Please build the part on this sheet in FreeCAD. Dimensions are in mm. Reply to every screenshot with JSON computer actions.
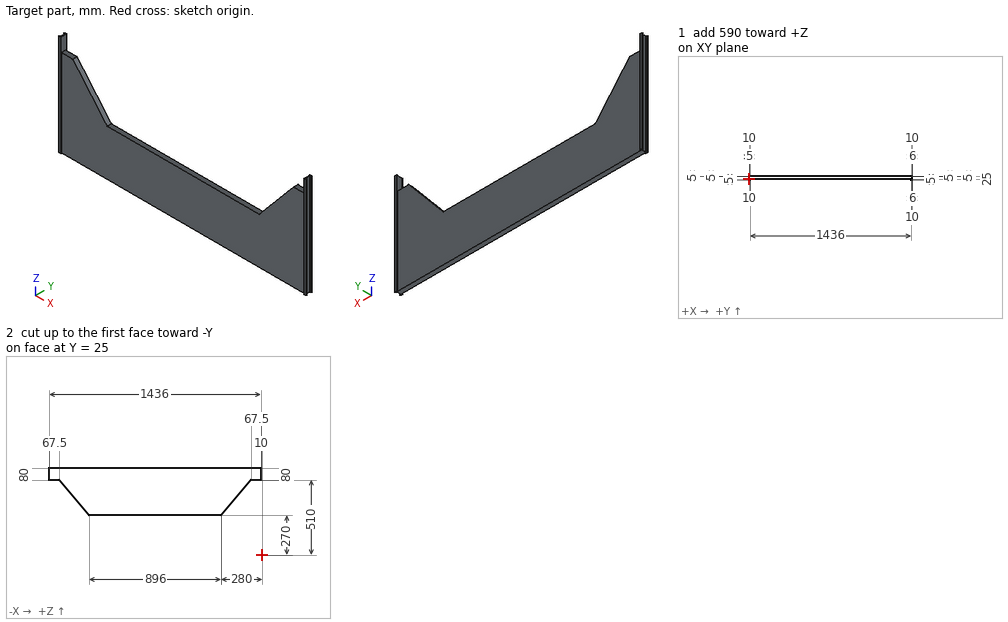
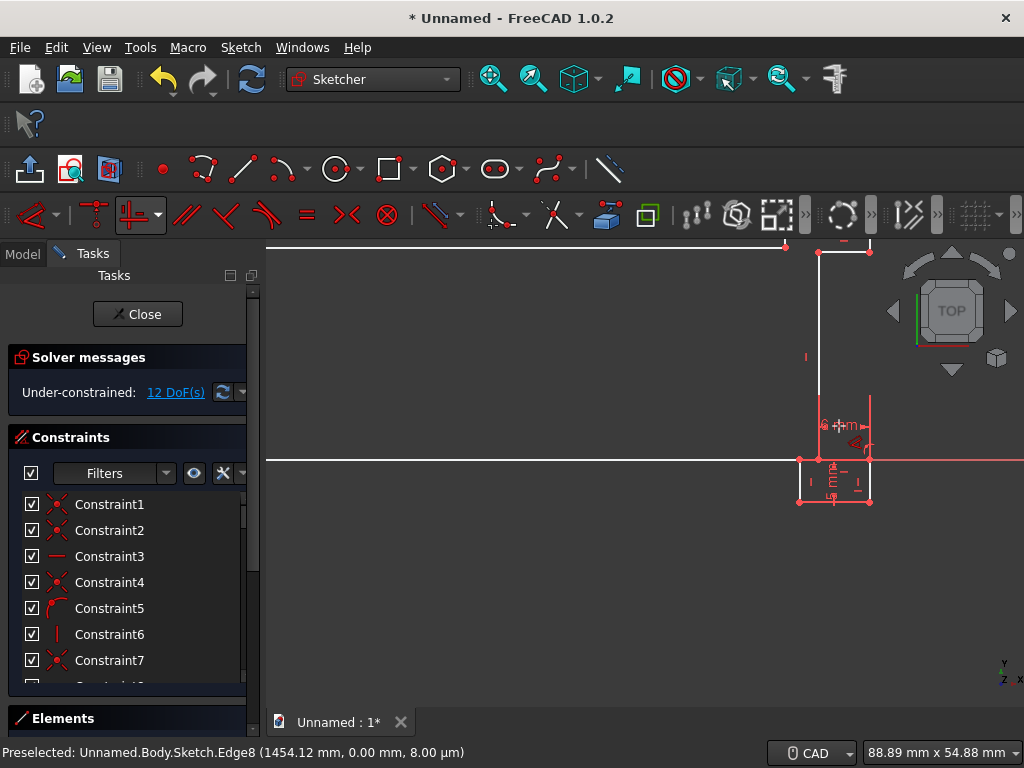
{"action": "scroll", "coordinate": [828, 478], "scroll_direction": "down", "scroll_amount": 16}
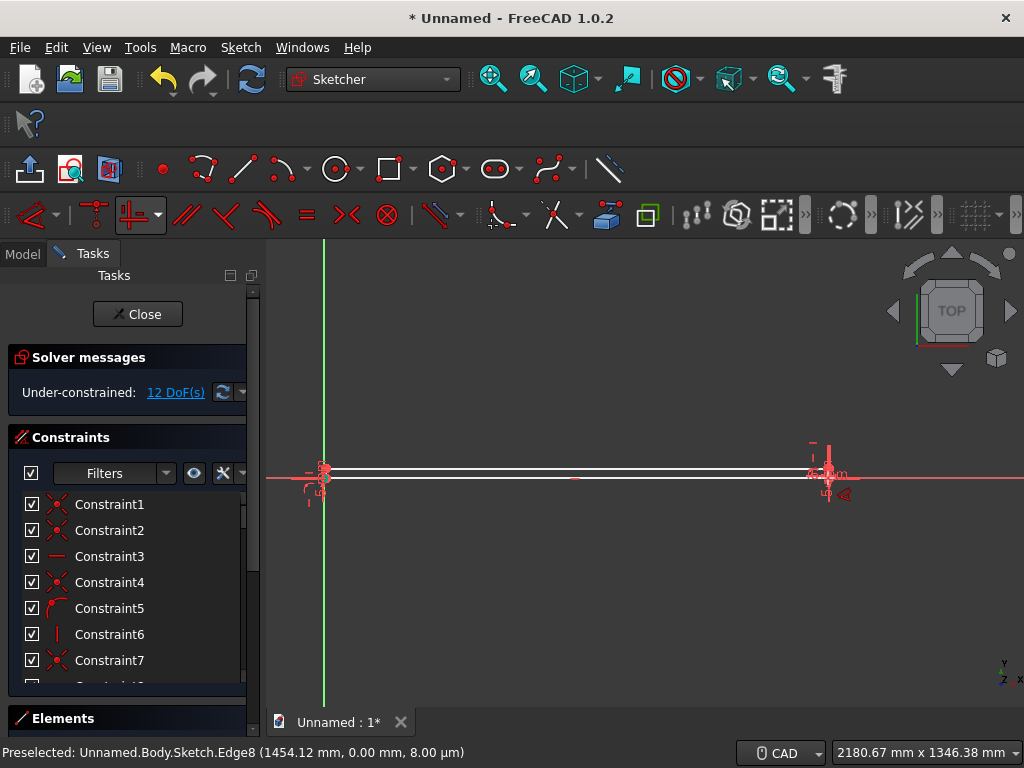
{"action": "scroll", "coordinate": [829, 469], "scroll_direction": "up", "scroll_amount": 15}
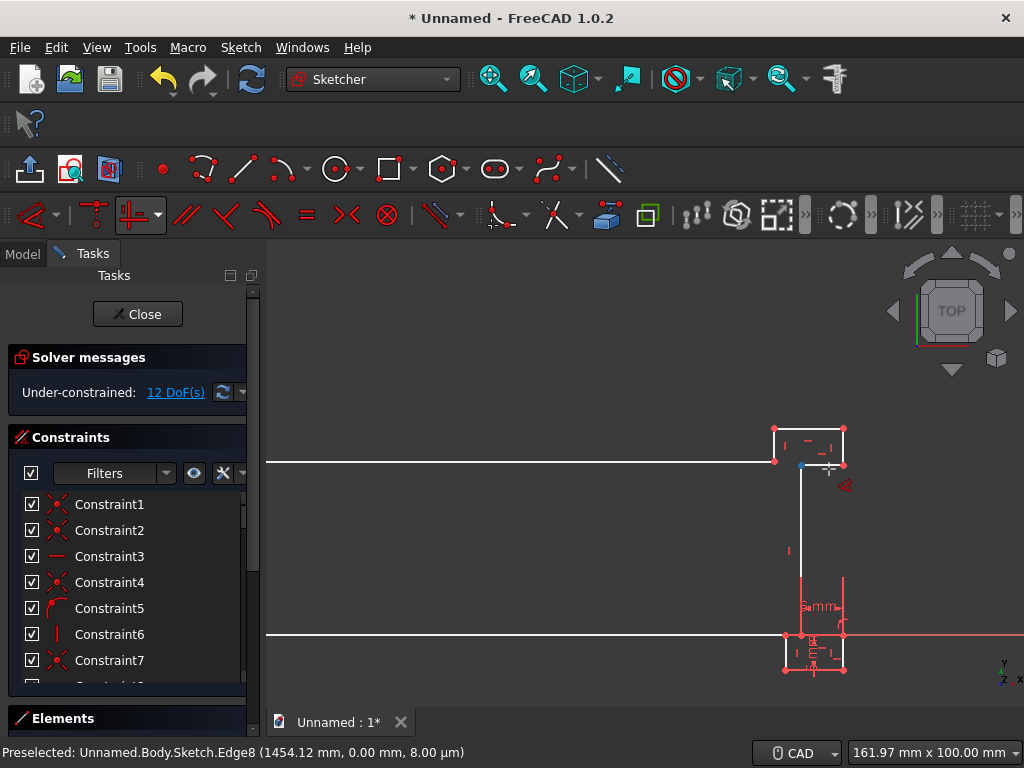
{"action": "left_click", "coordinate": [814, 465]}
{"action": "left_click", "coordinate": [822, 499]}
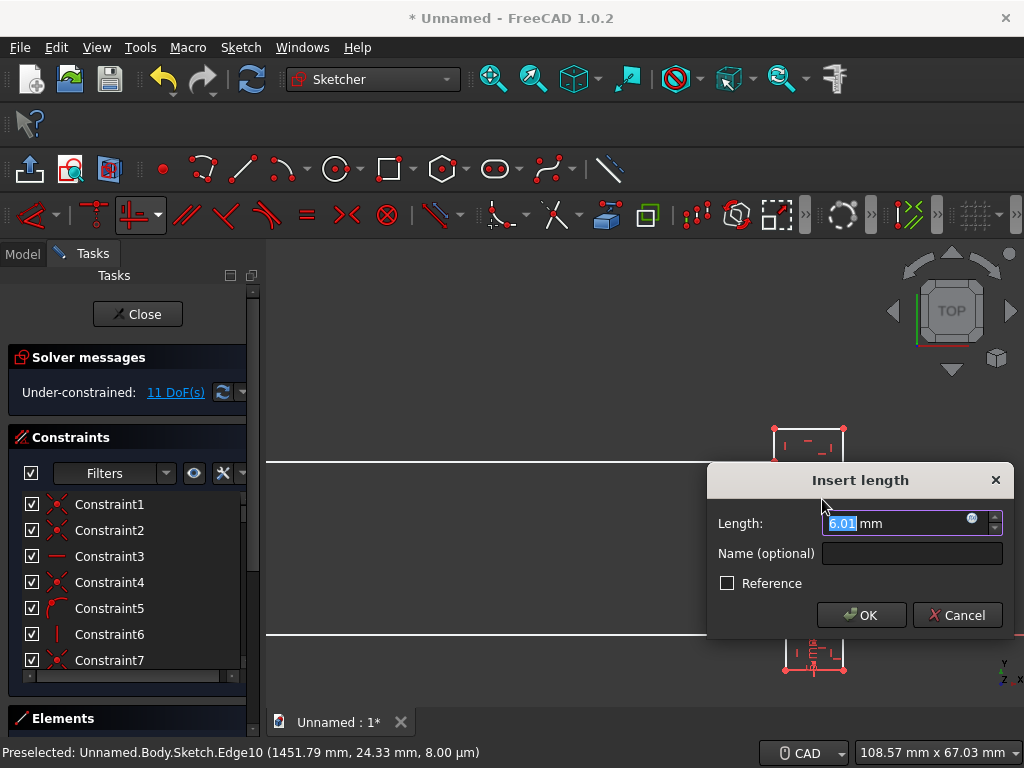
{"action": "type", "text": "6"}
{"action": "key", "text": "Return"}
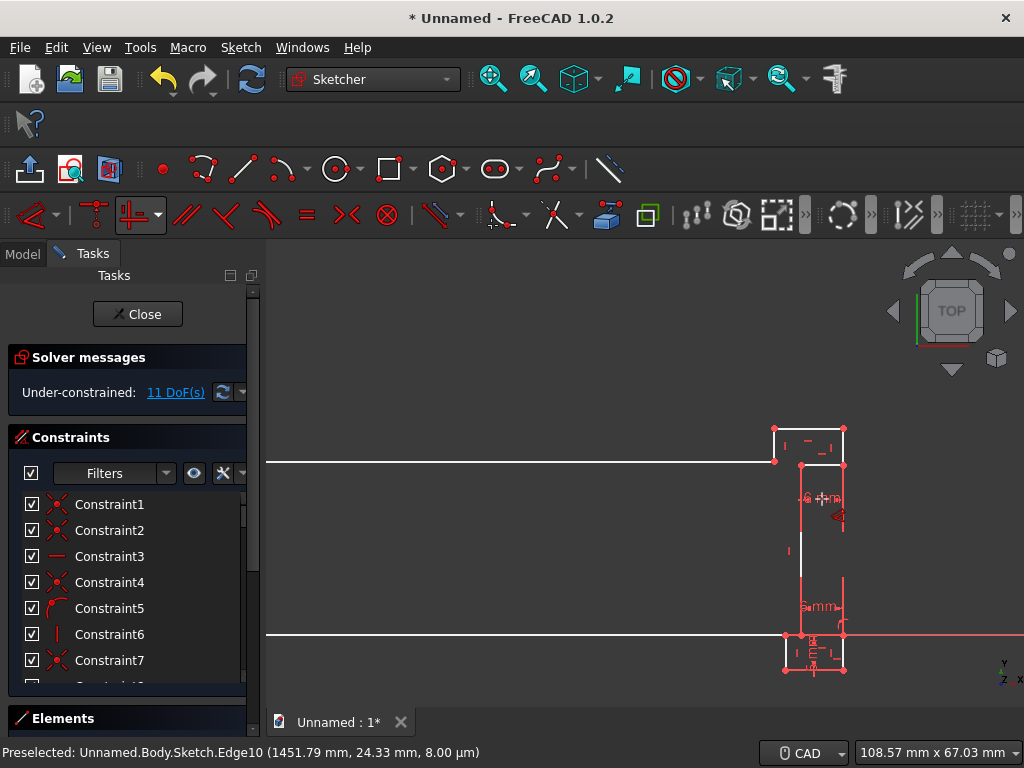
{"action": "left_click", "coordinate": [843, 454]}
{"action": "left_click", "coordinate": [809, 447]}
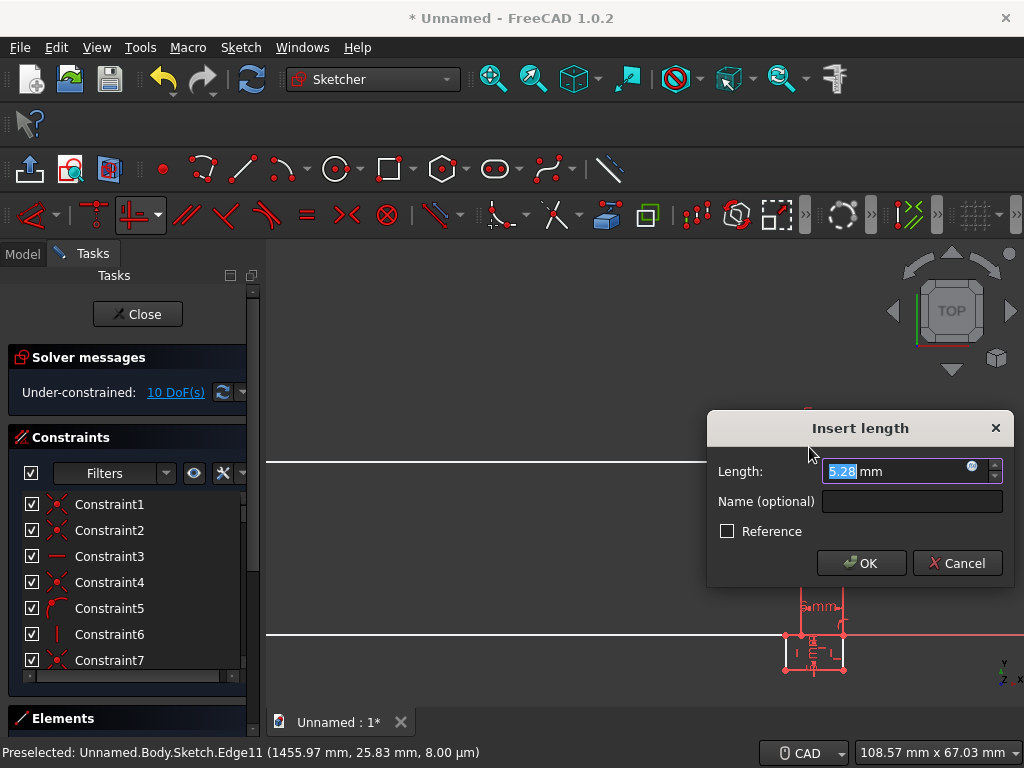
{"action": "type", "text": "5"}
{"action": "key", "text": "Return"}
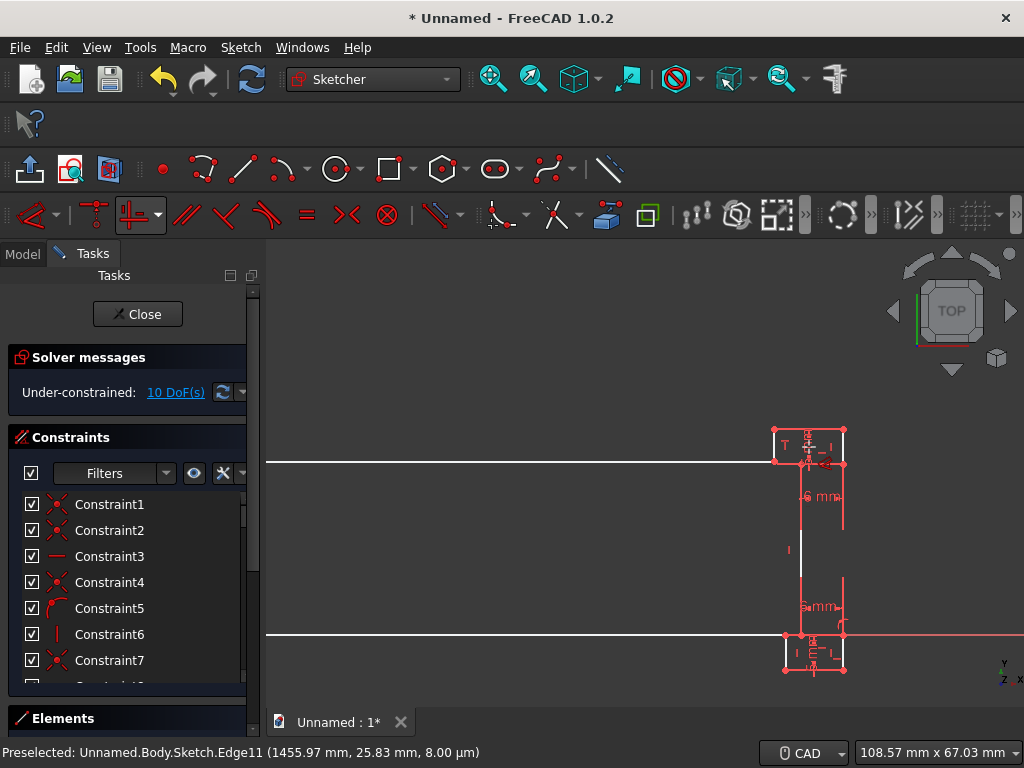
{"action": "left_click", "coordinate": [774, 439]}
{"action": "left_click", "coordinate": [716, 445]}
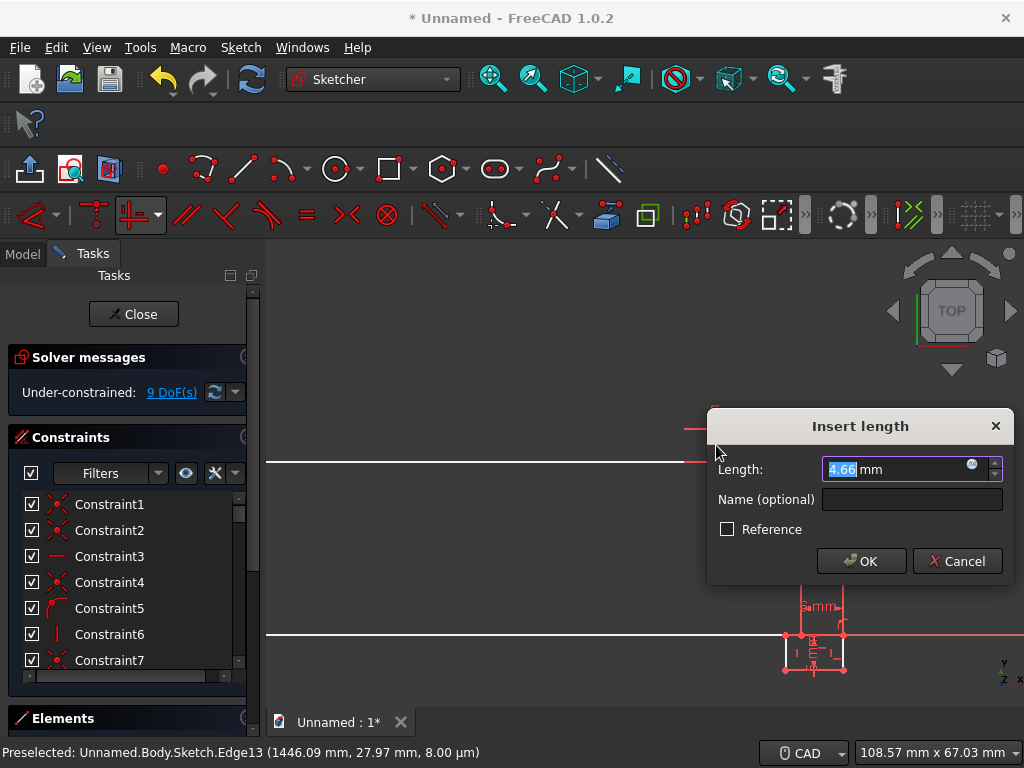
{"action": "type", "text": "5"}
{"action": "key", "text": "Return"}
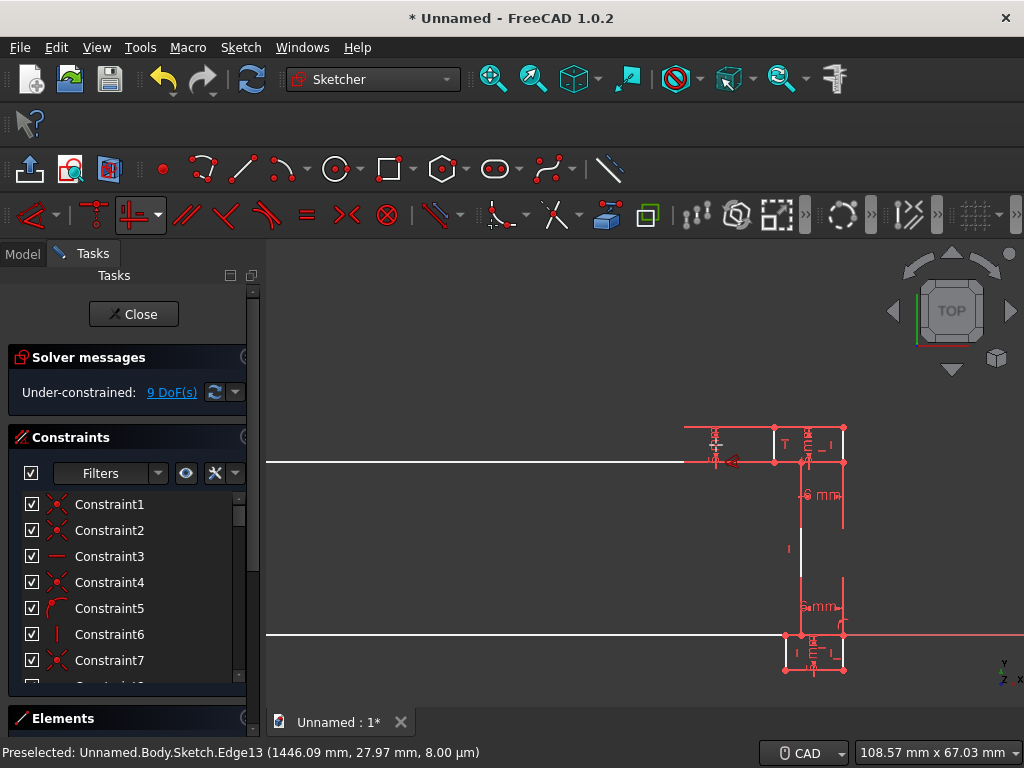
{"action": "scroll", "coordinate": [829, 469], "scroll_direction": "down", "scroll_amount": 15}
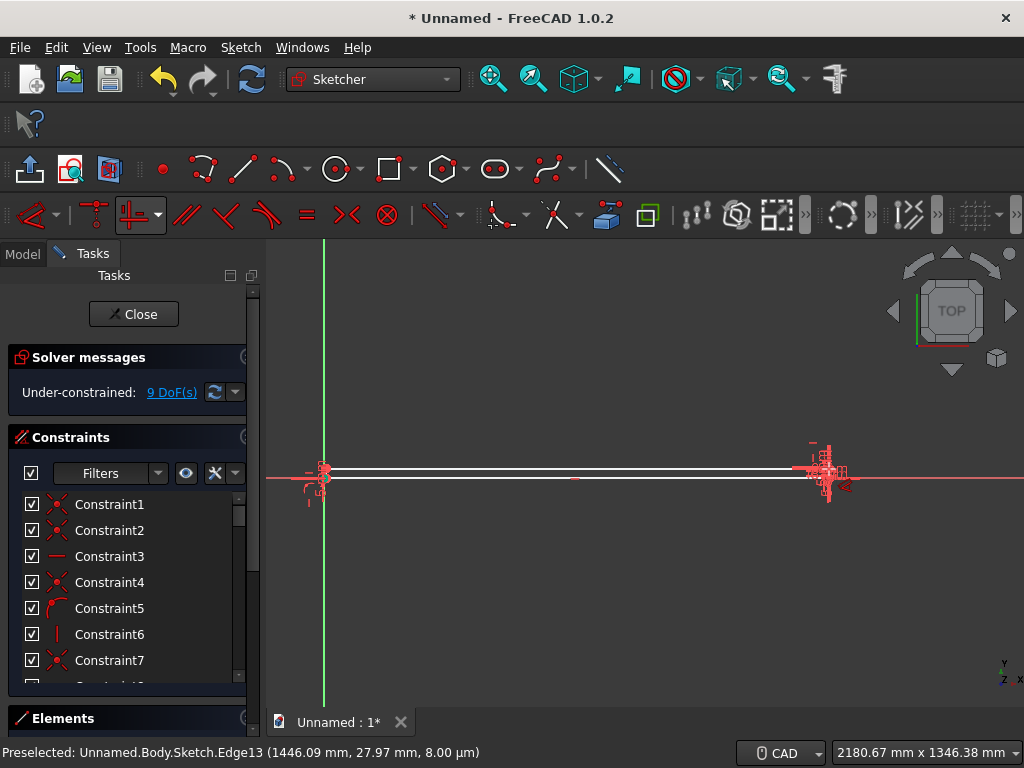
{"action": "scroll", "coordinate": [328, 469], "scroll_direction": "up", "scroll_amount": 16}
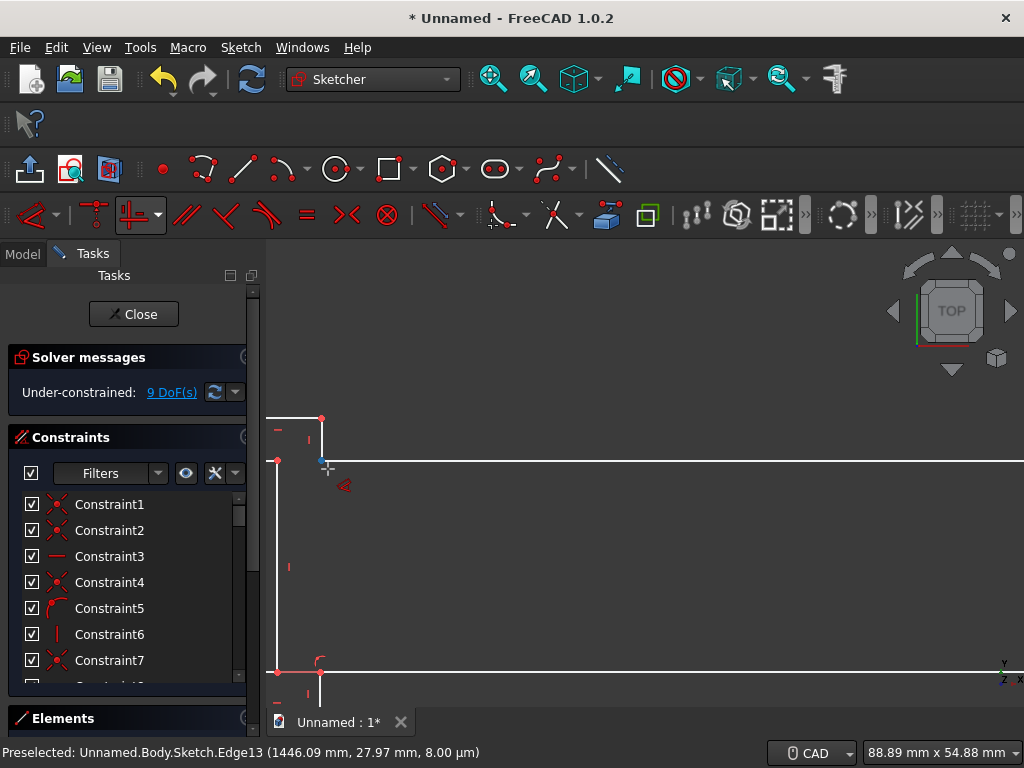
{"action": "left_click", "coordinate": [322, 448]}
{"action": "left_click", "coordinate": [356, 439]}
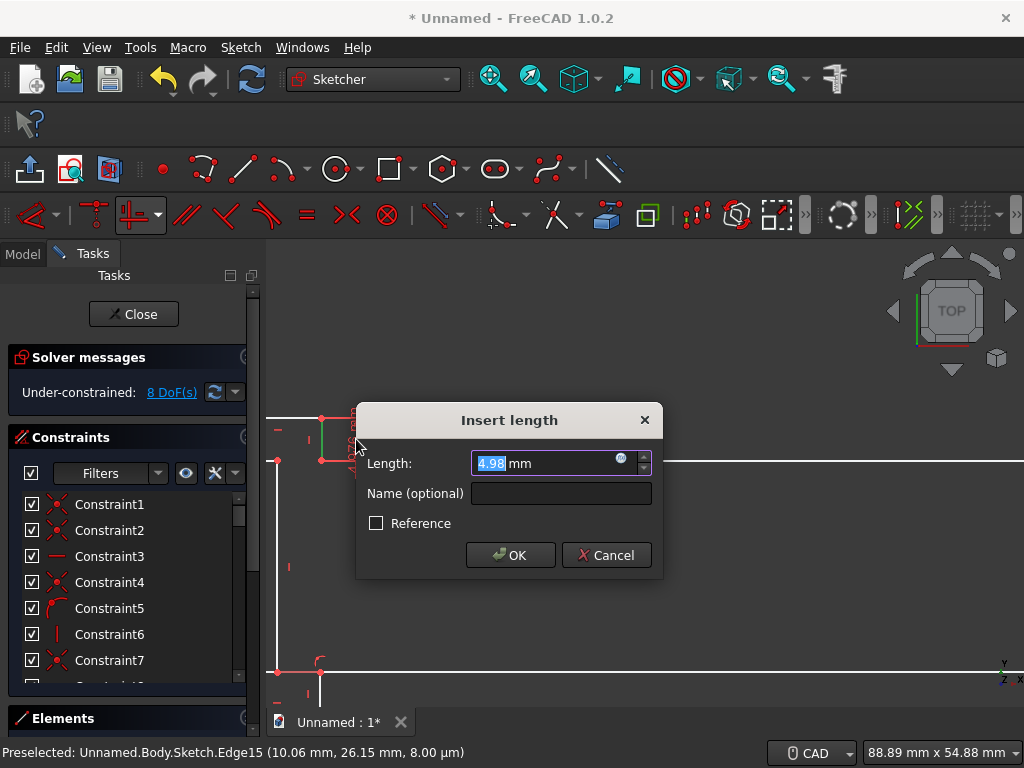
{"action": "type", "text": "5"}
{"action": "key", "text": "Return"}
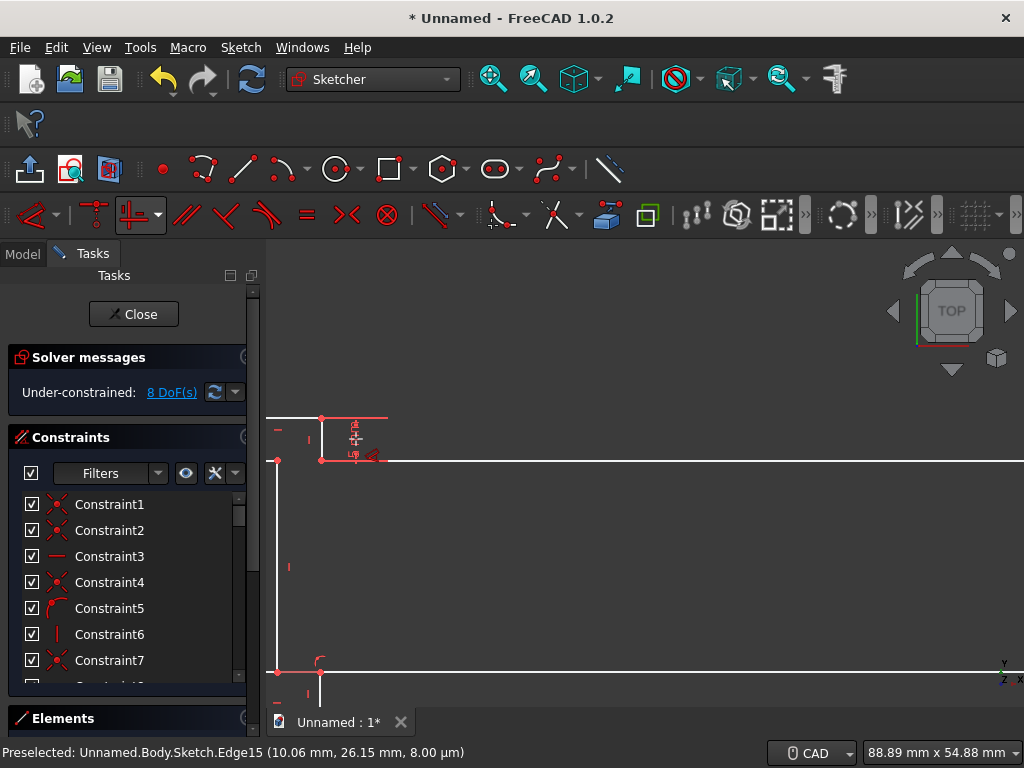
{"action": "scroll", "coordinate": [327, 469], "scroll_direction": "down", "scroll_amount": 16}